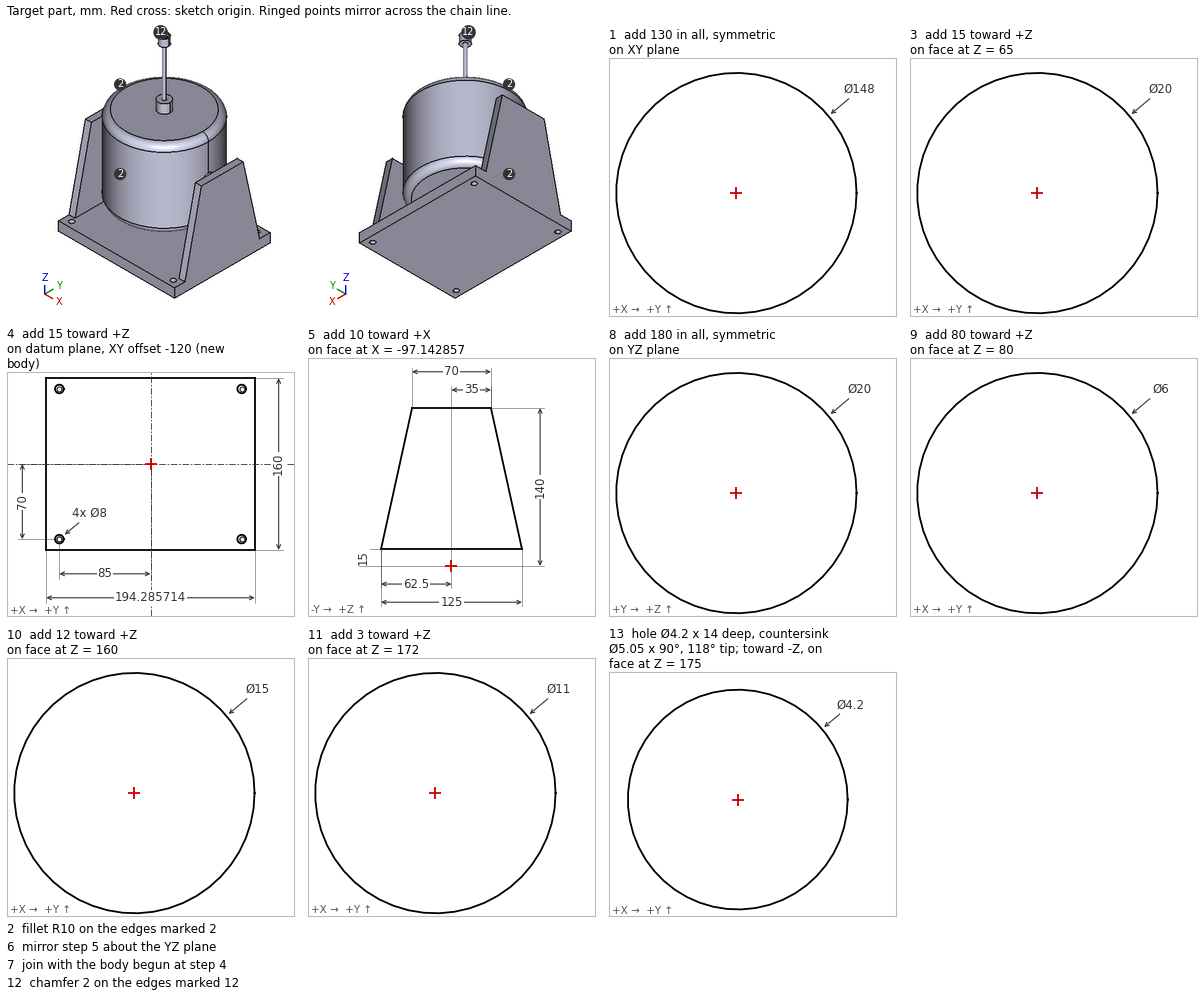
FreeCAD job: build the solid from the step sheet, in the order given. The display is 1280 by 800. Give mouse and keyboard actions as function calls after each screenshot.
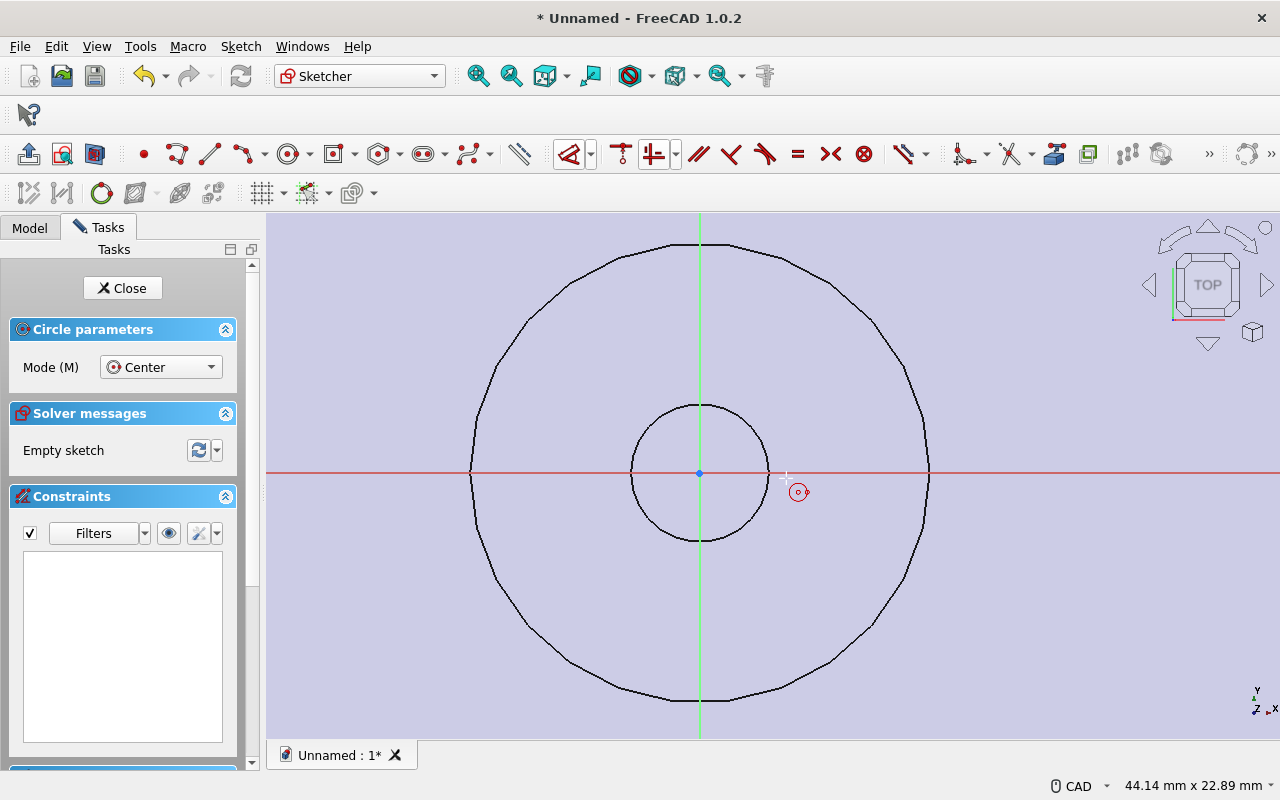
click(700, 473)
click(822, 351)
key(Escape)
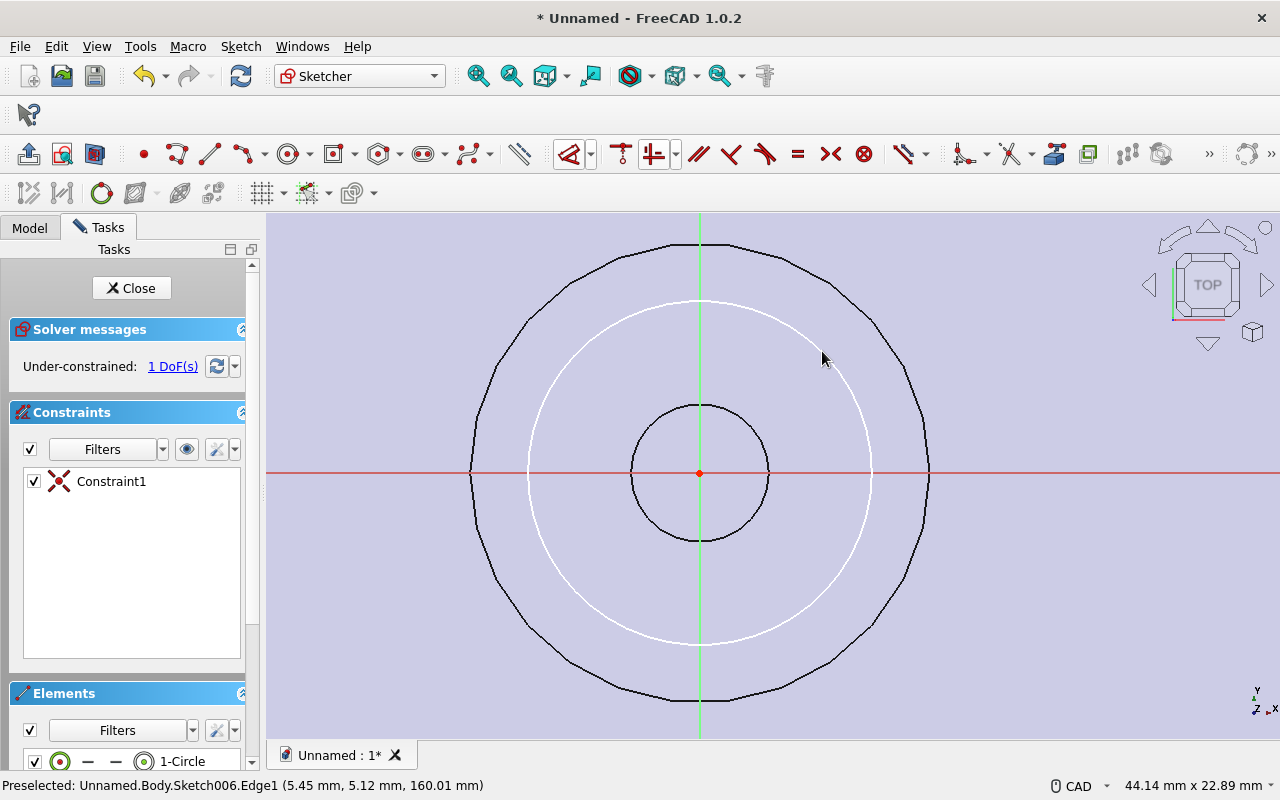
click(821, 351)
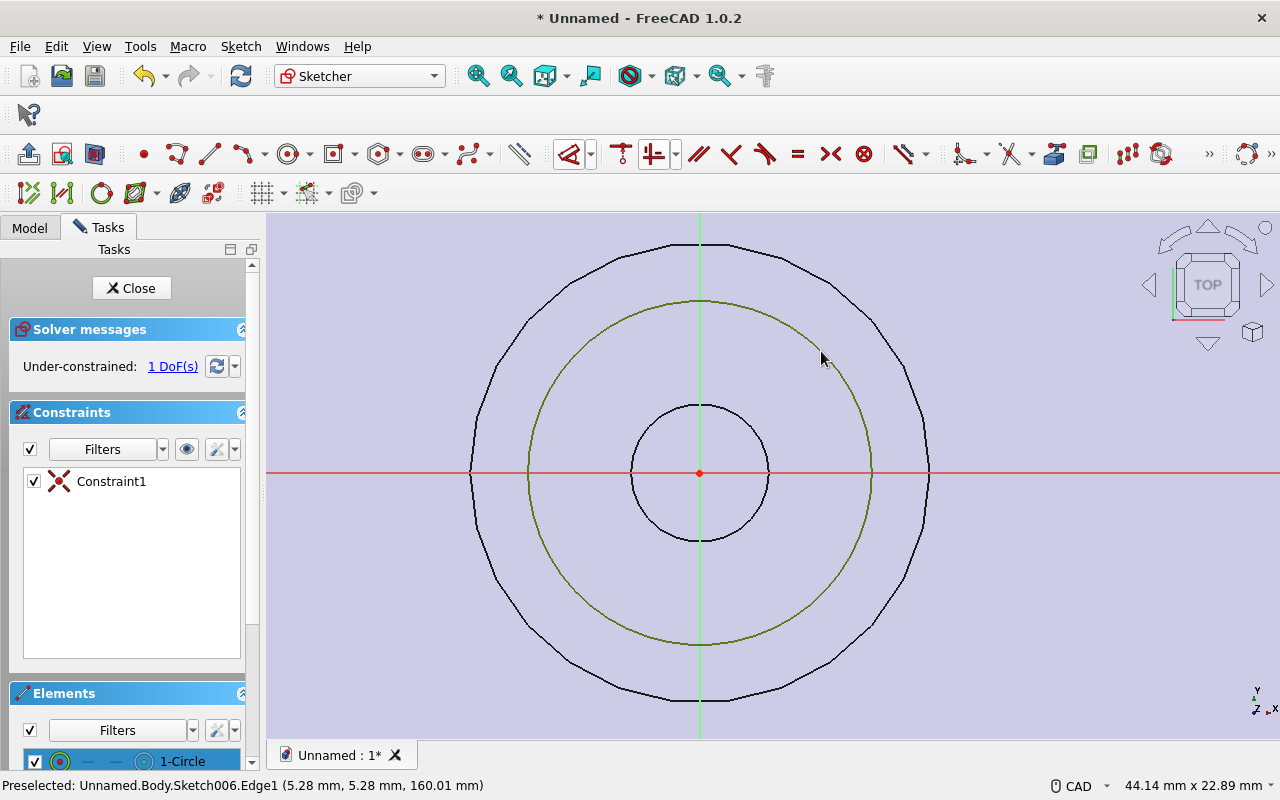
key(k)
key(o)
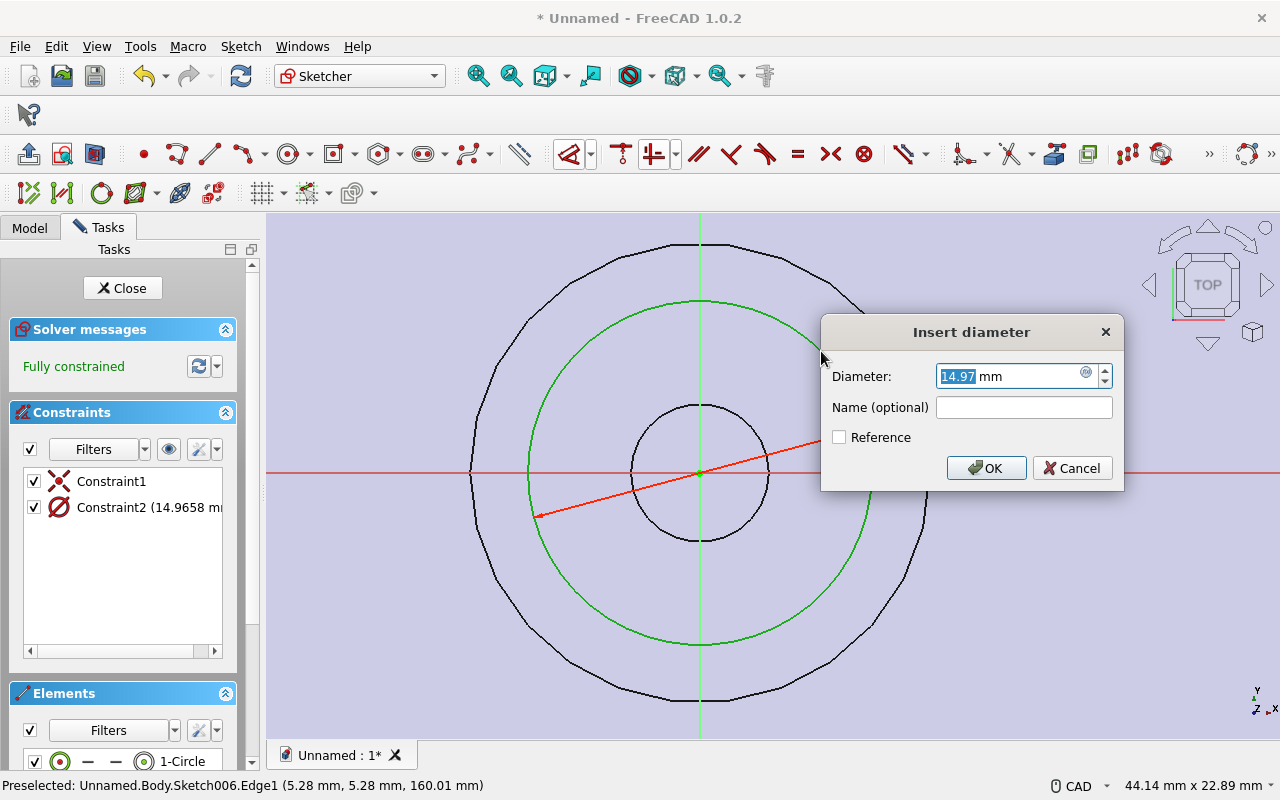
text(15)
key(Return)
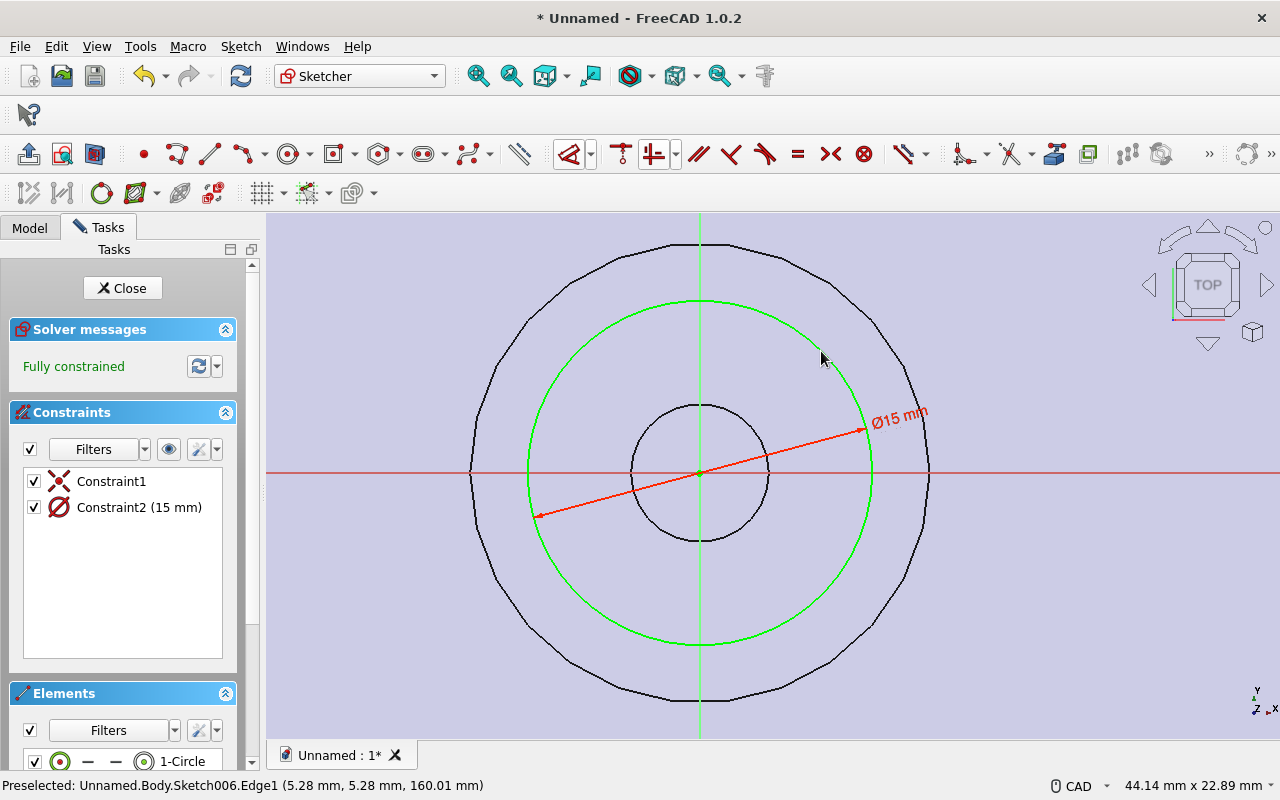
click(123, 288)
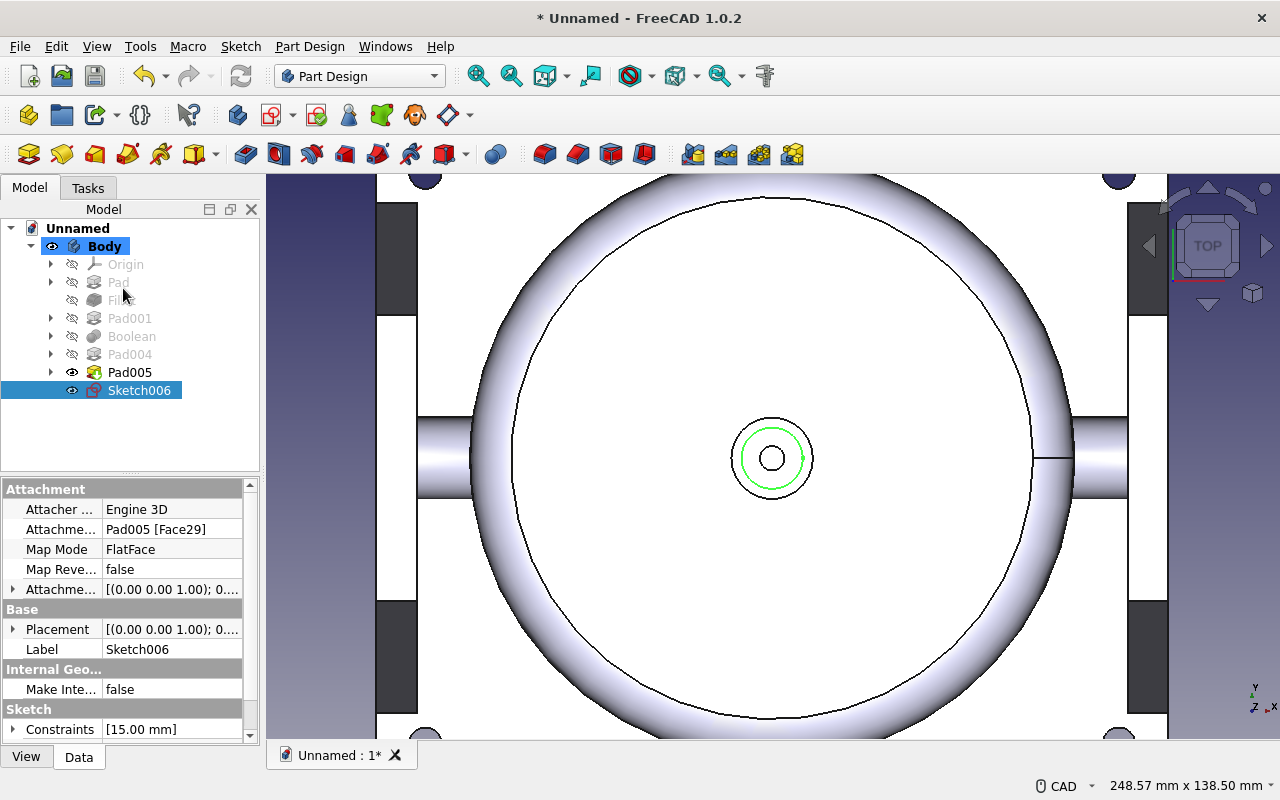
click(29, 154)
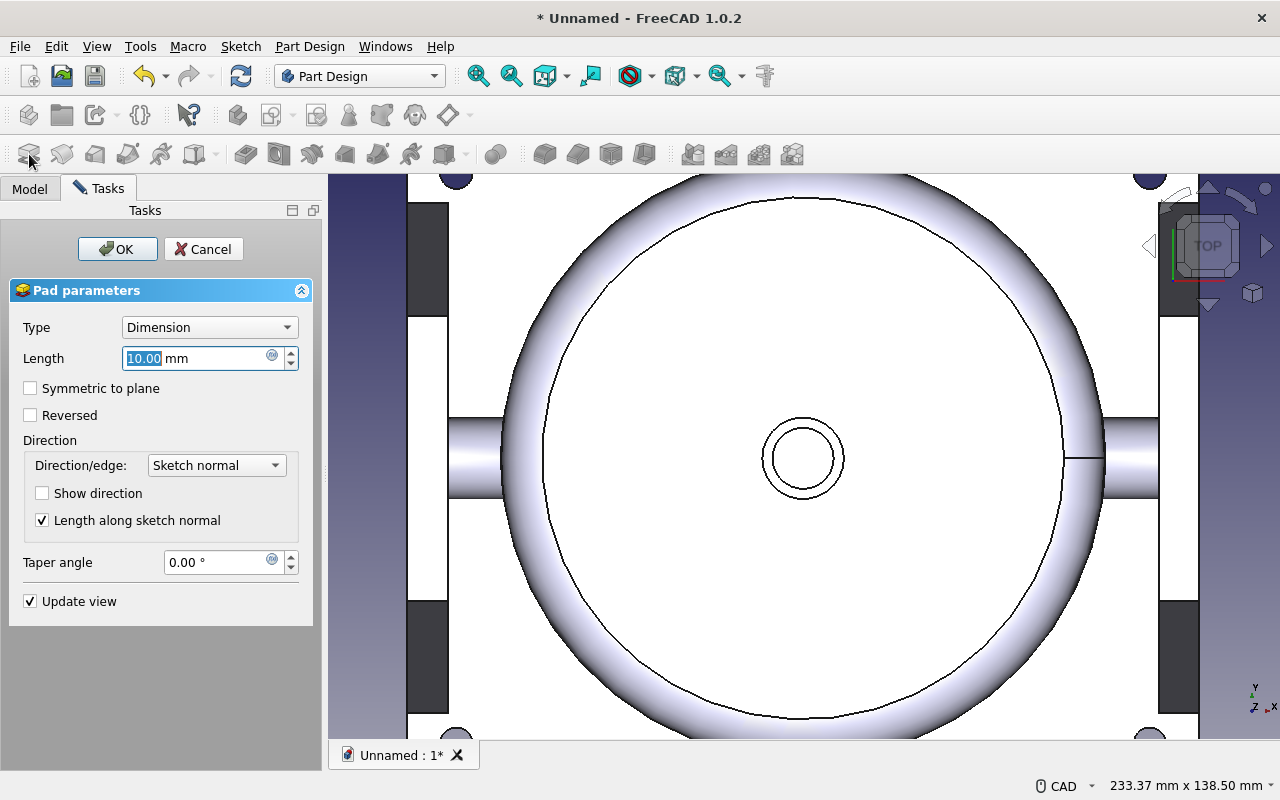
text(12)
key(Tab)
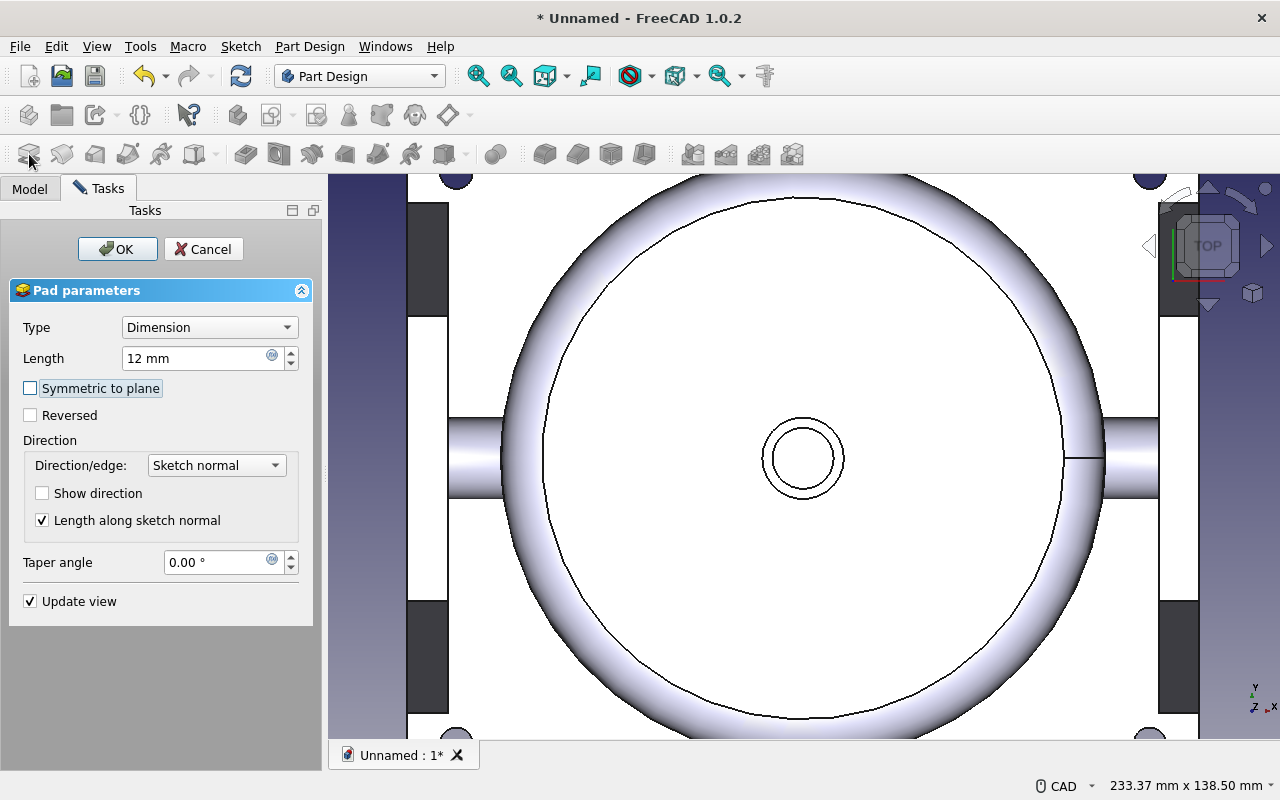
click(118, 249)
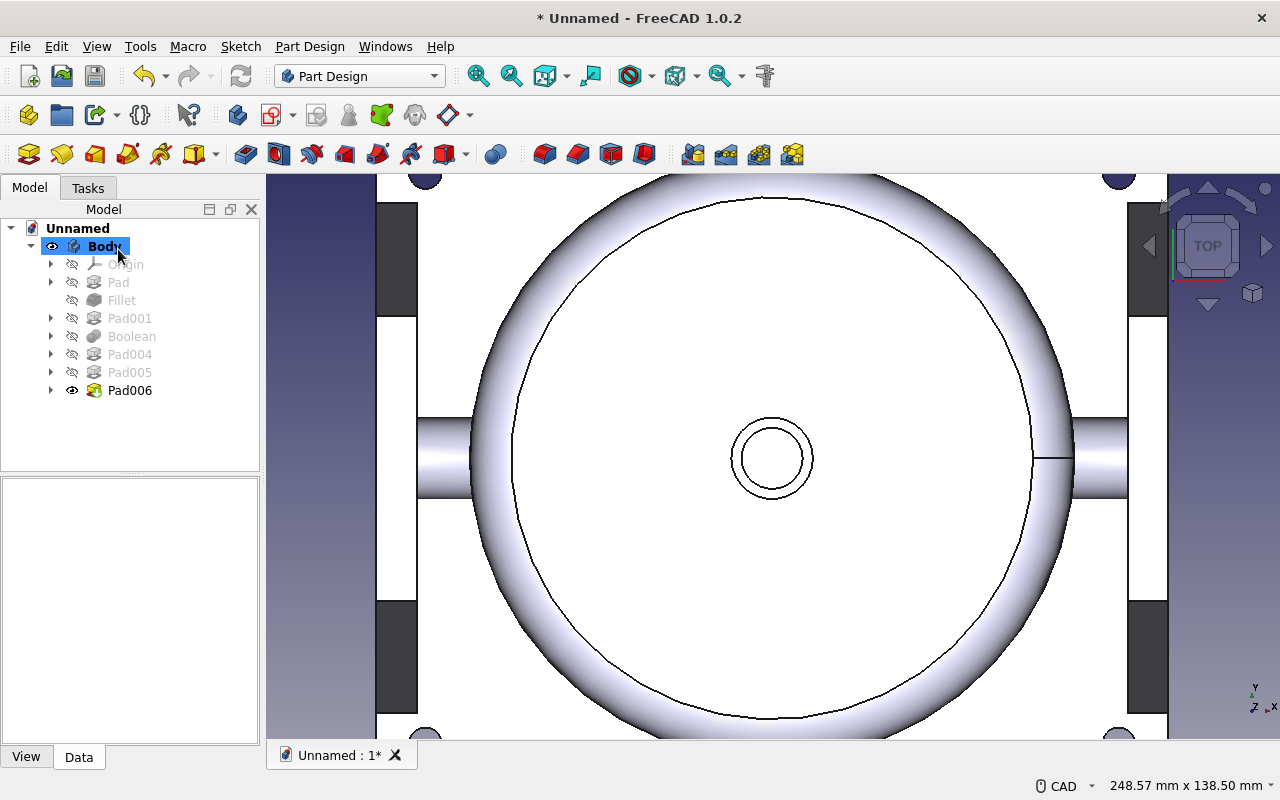
click(479, 76)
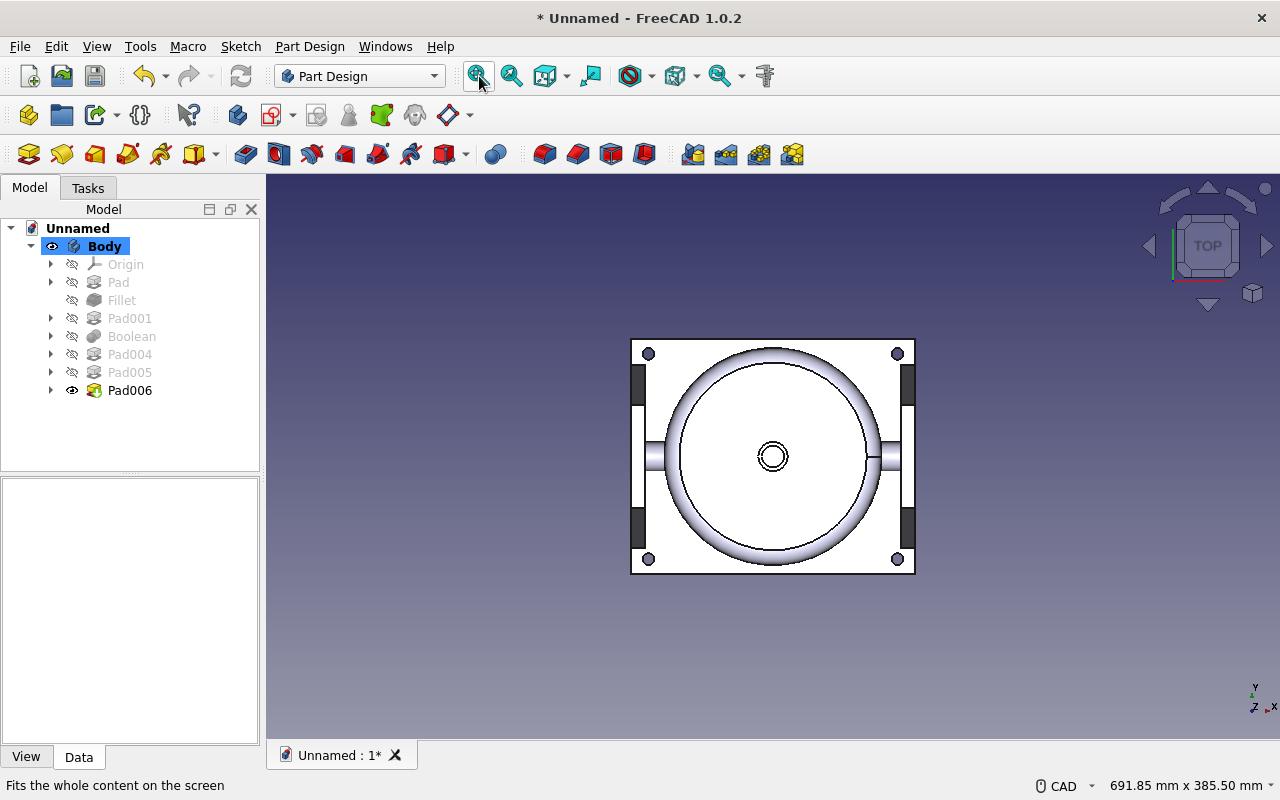
click(773, 455)